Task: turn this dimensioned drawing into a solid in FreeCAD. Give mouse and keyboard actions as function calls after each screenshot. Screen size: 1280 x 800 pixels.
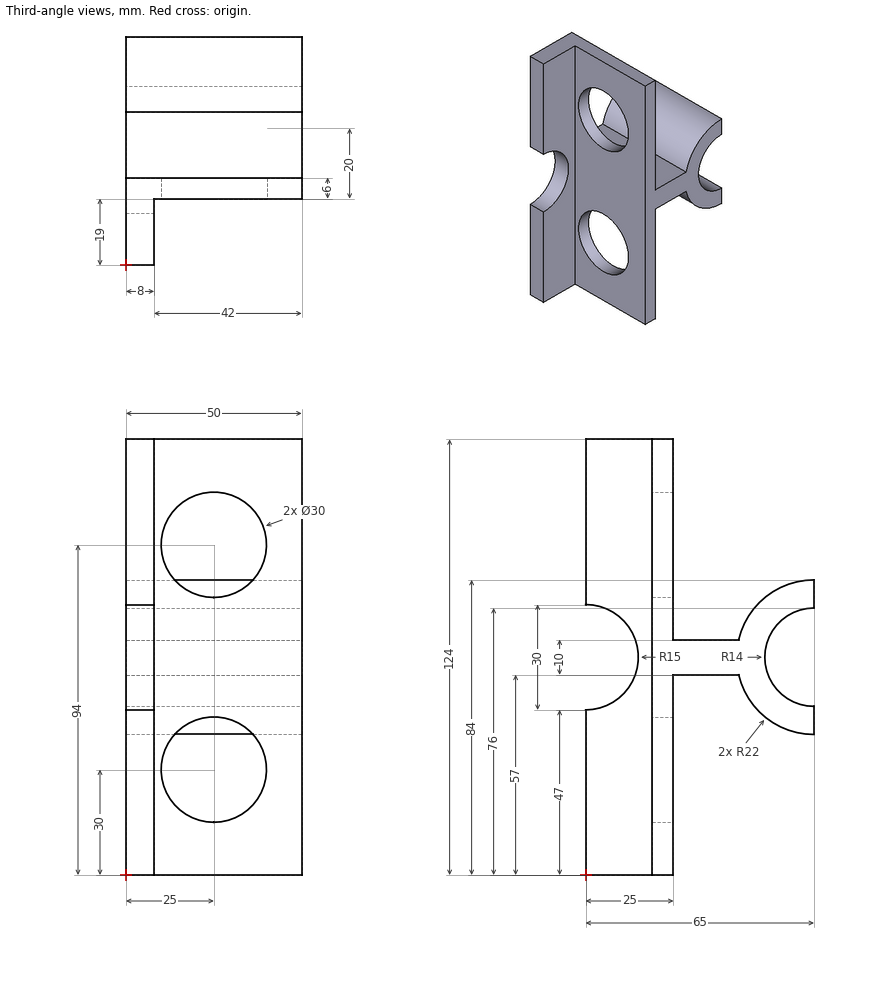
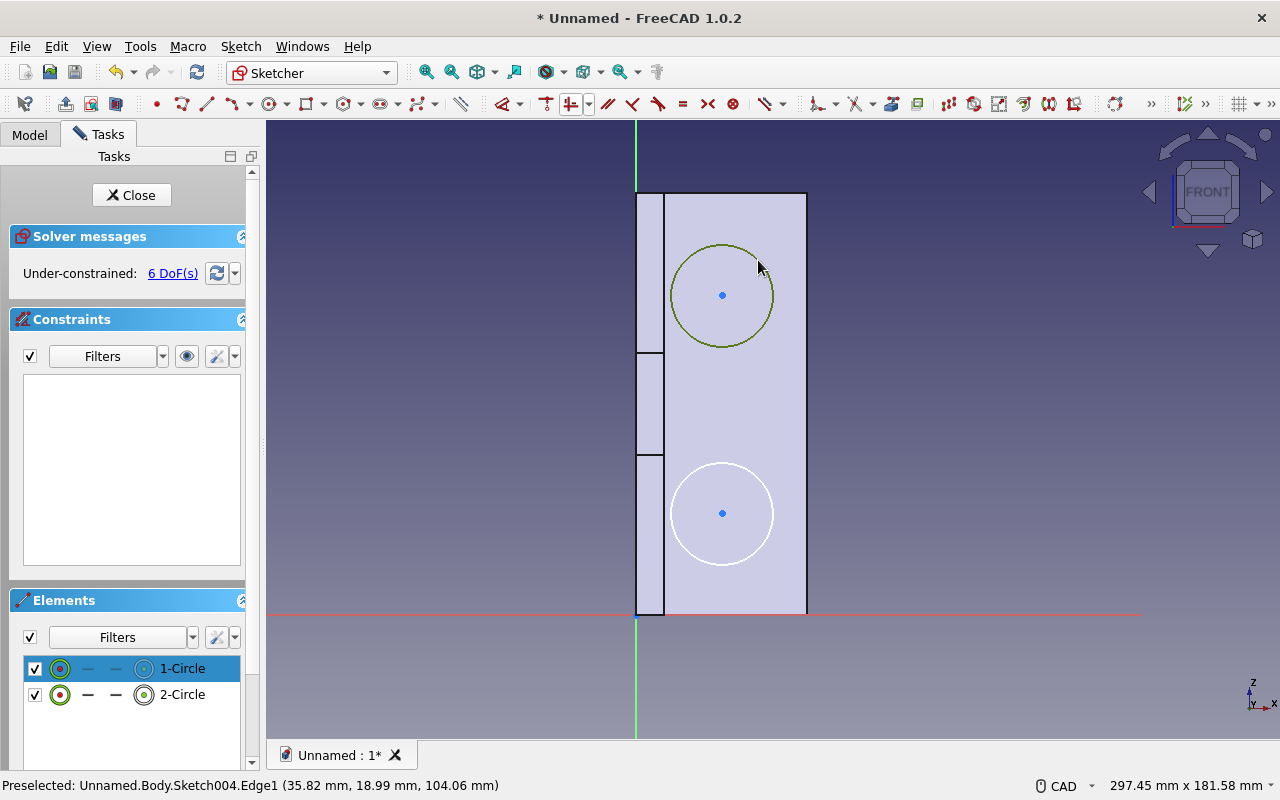
click(758, 478)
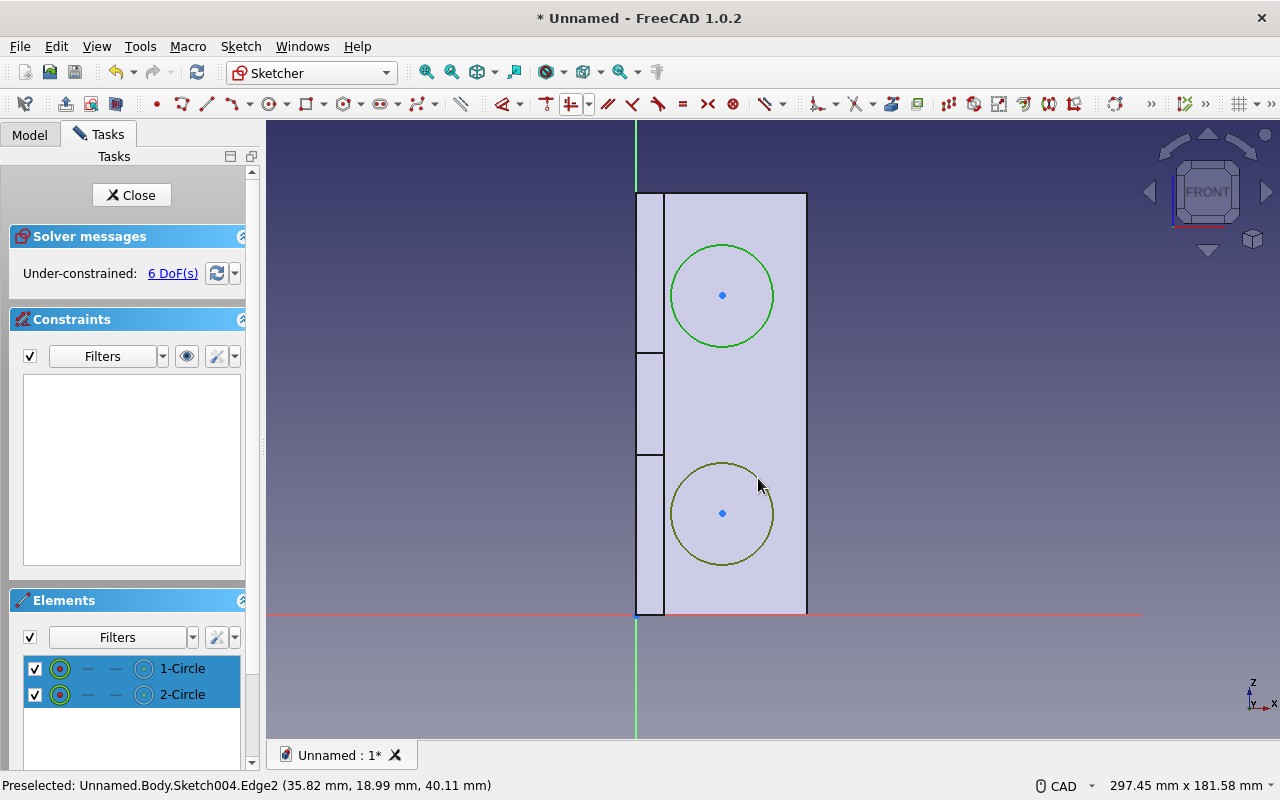
key(e)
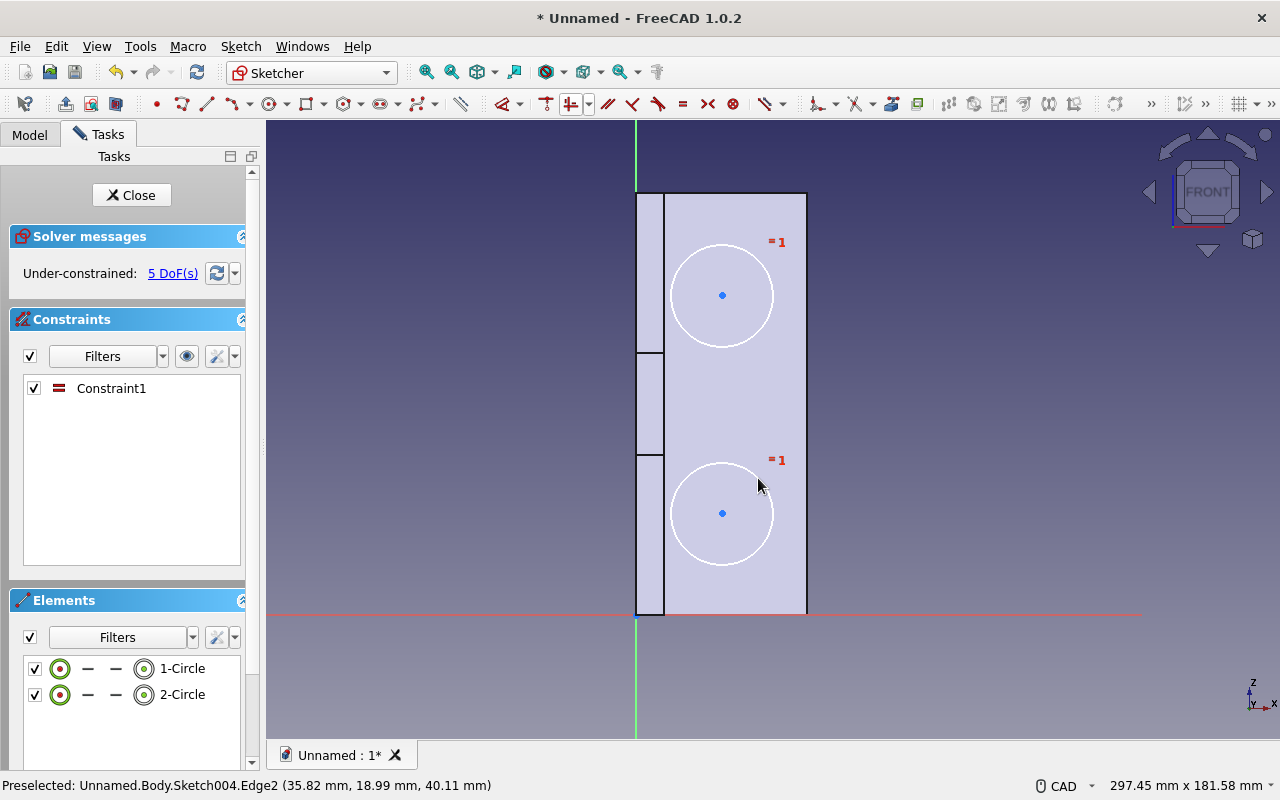
click(722, 296)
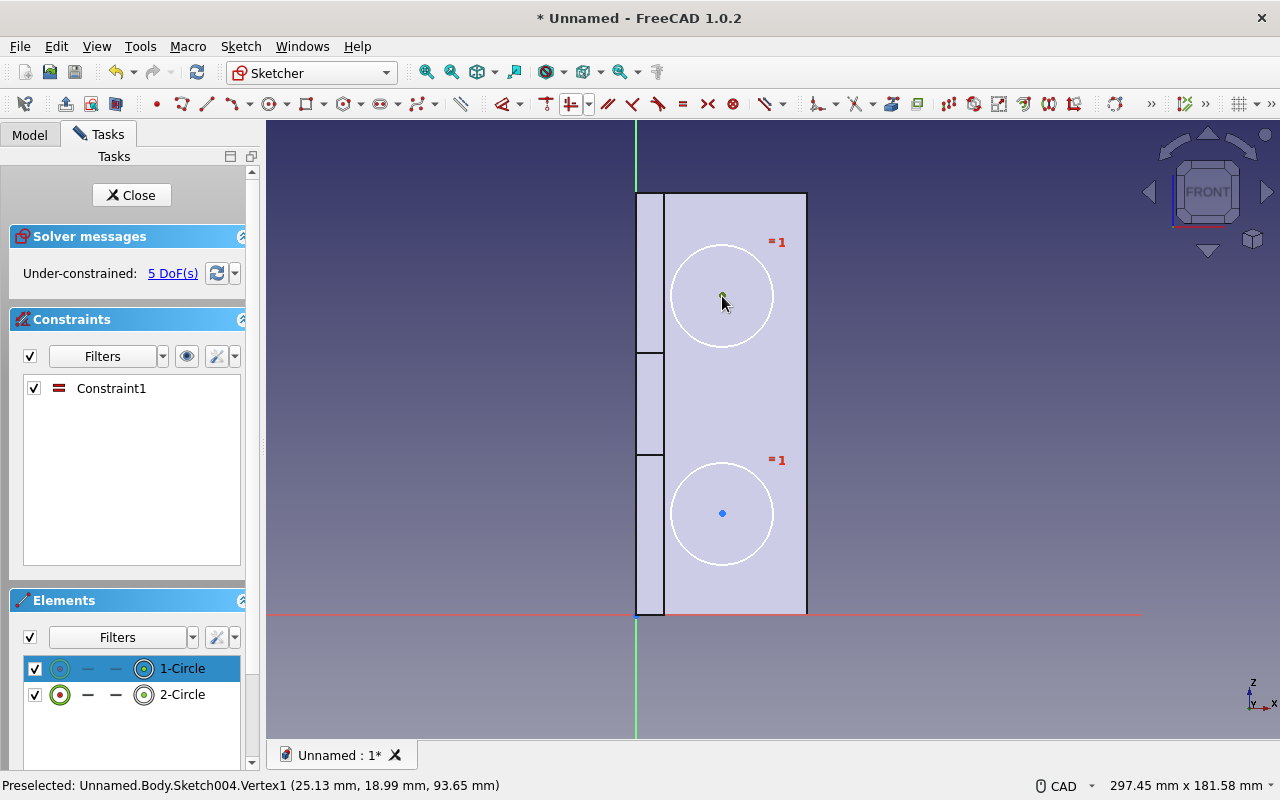
click(722, 514)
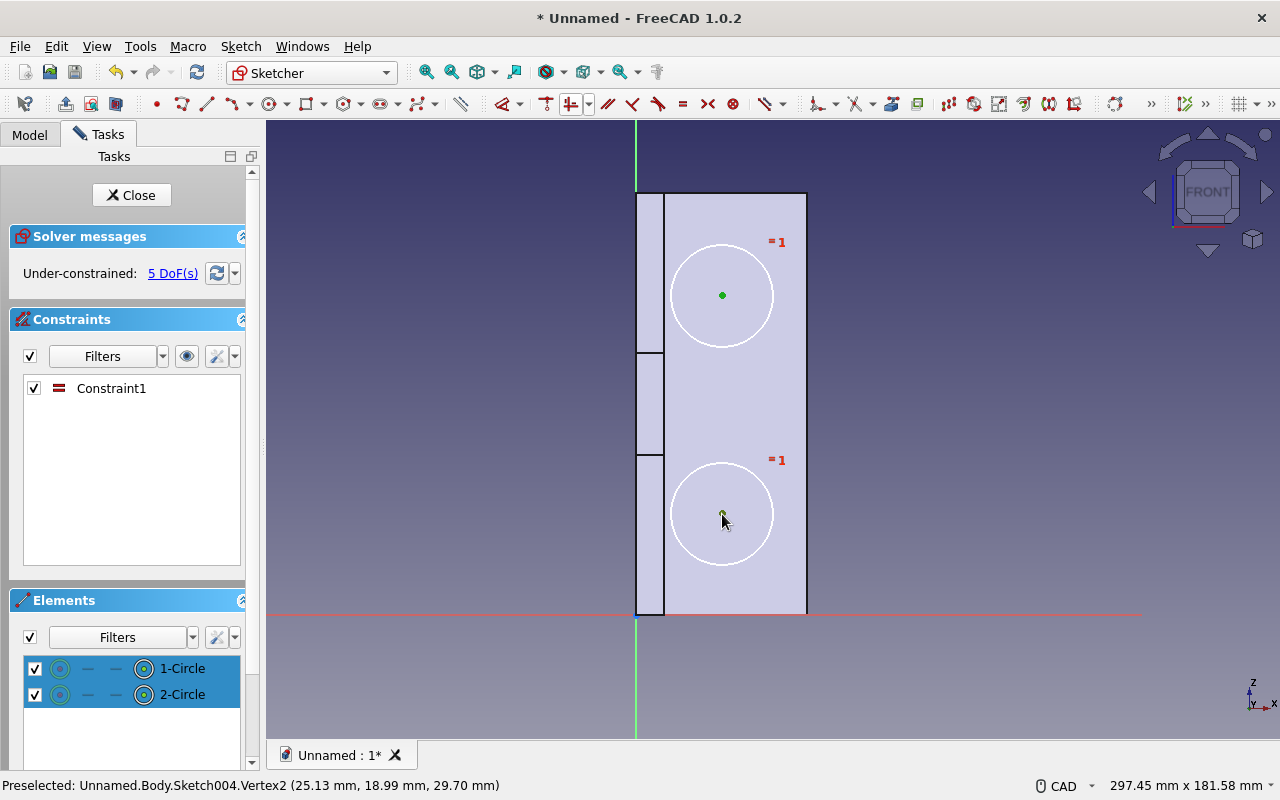
key(v)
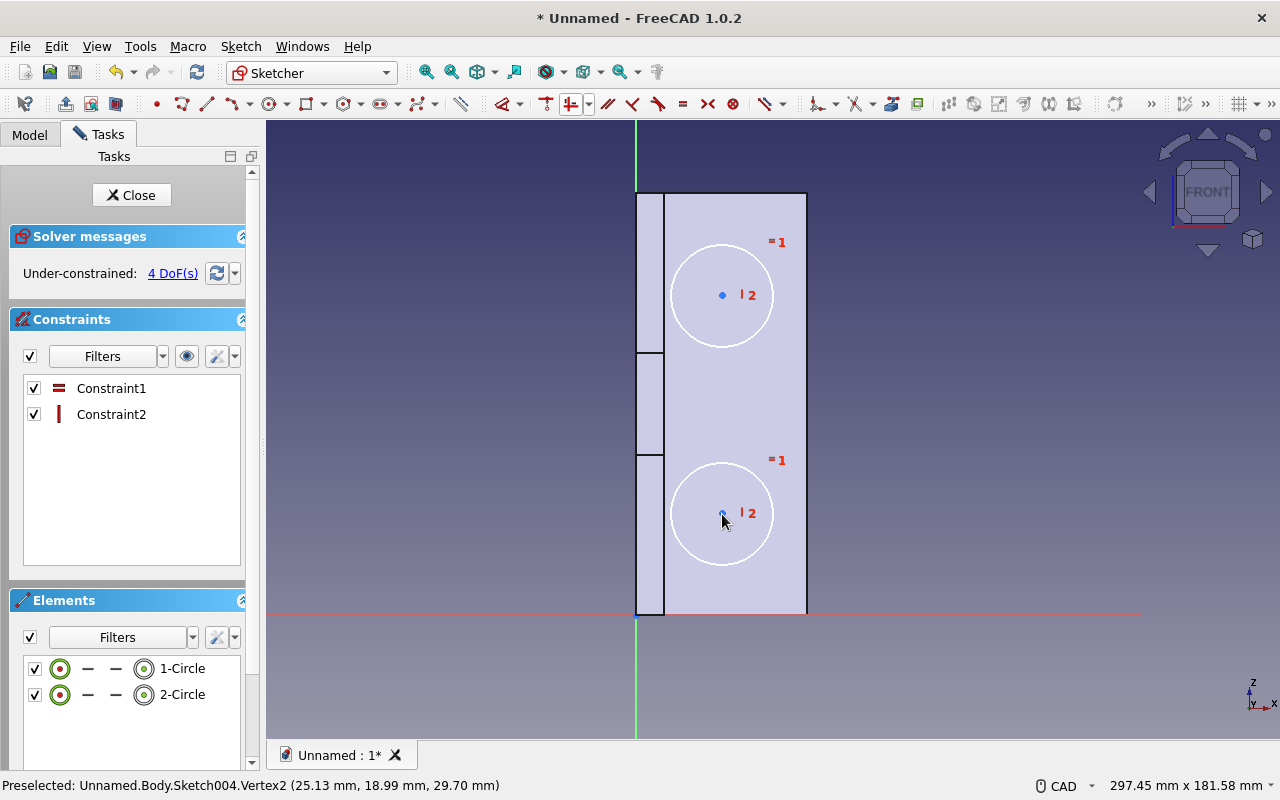
key(d)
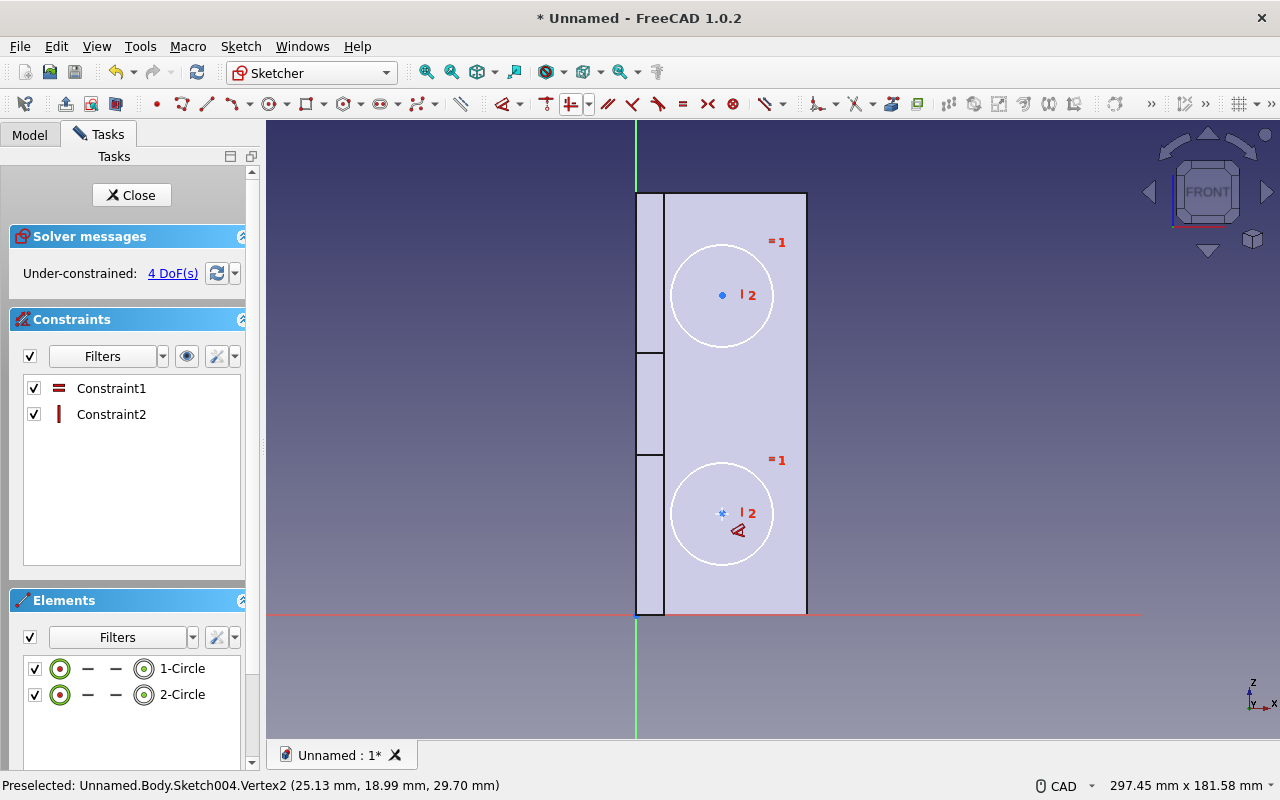
click(758, 260)
click(781, 237)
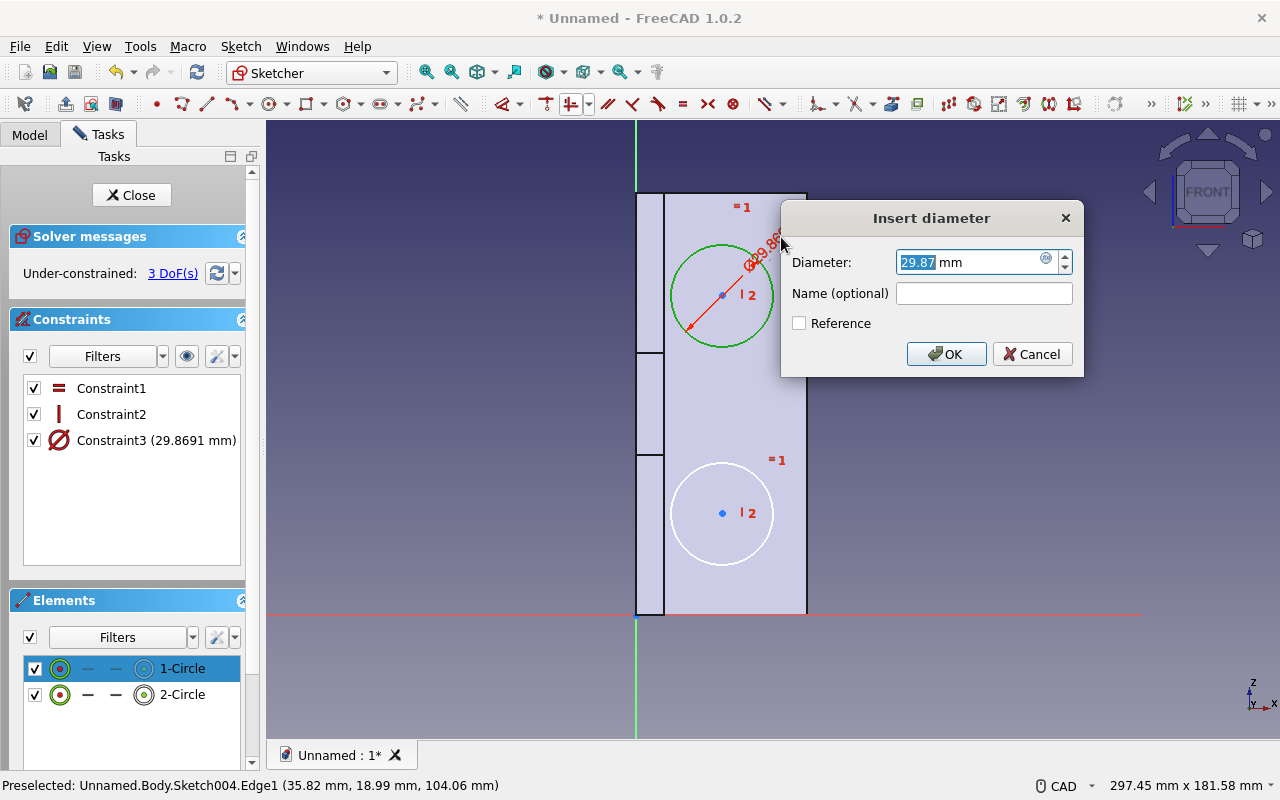
text(30)
key(Return)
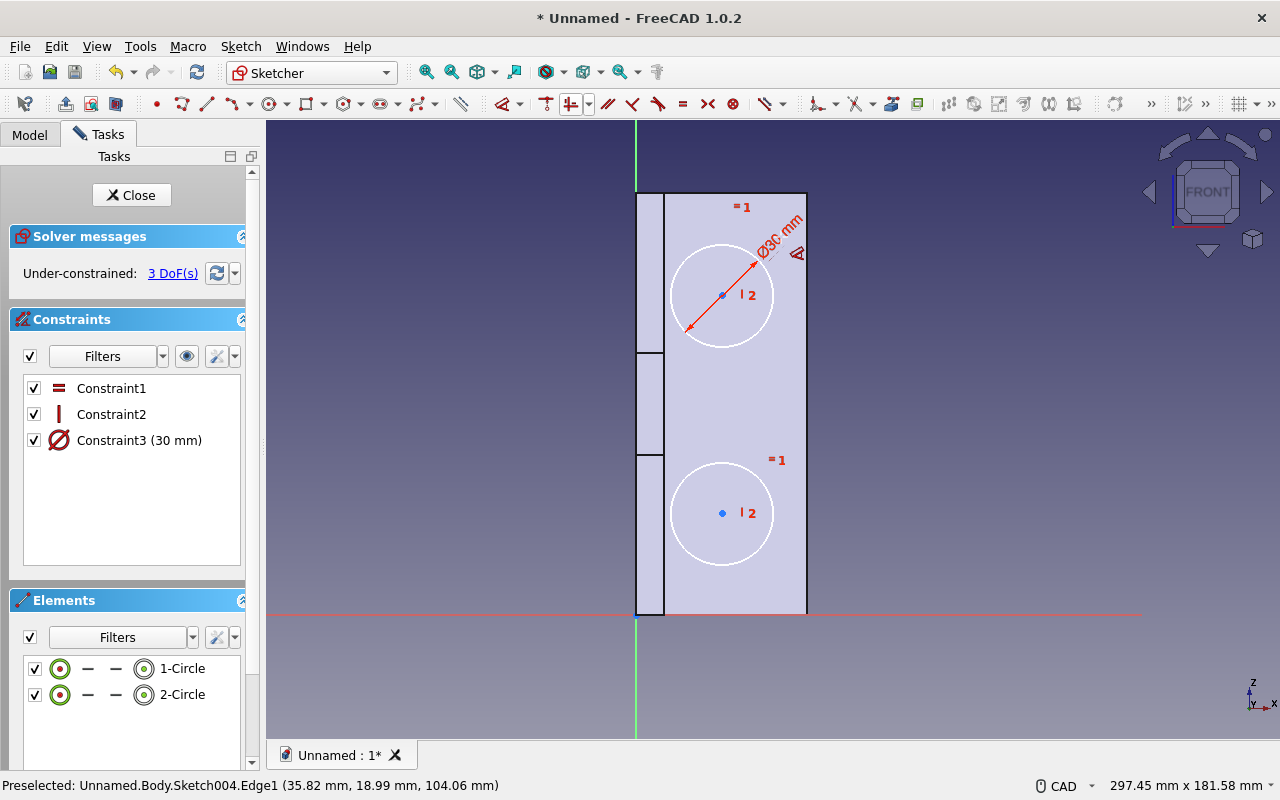
click(722, 296)
click(679, 649)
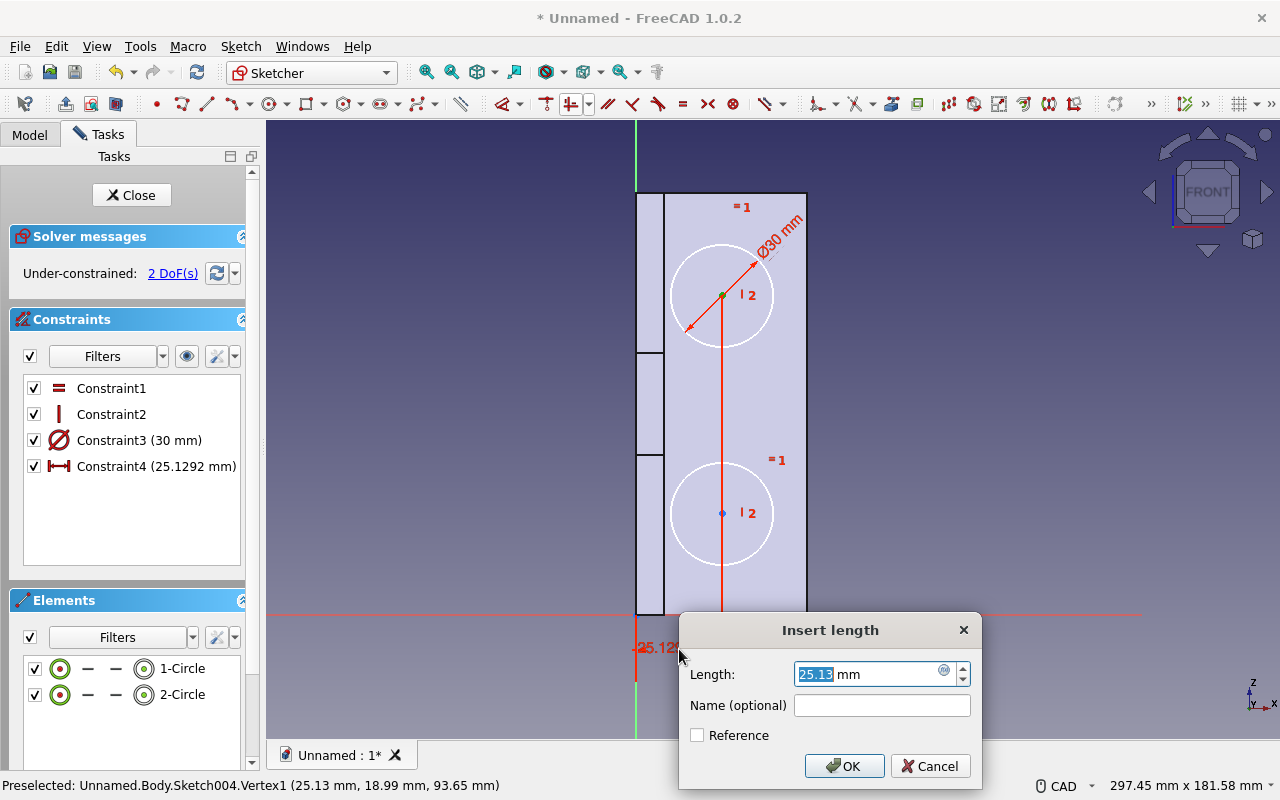
text(25)
key(Return)